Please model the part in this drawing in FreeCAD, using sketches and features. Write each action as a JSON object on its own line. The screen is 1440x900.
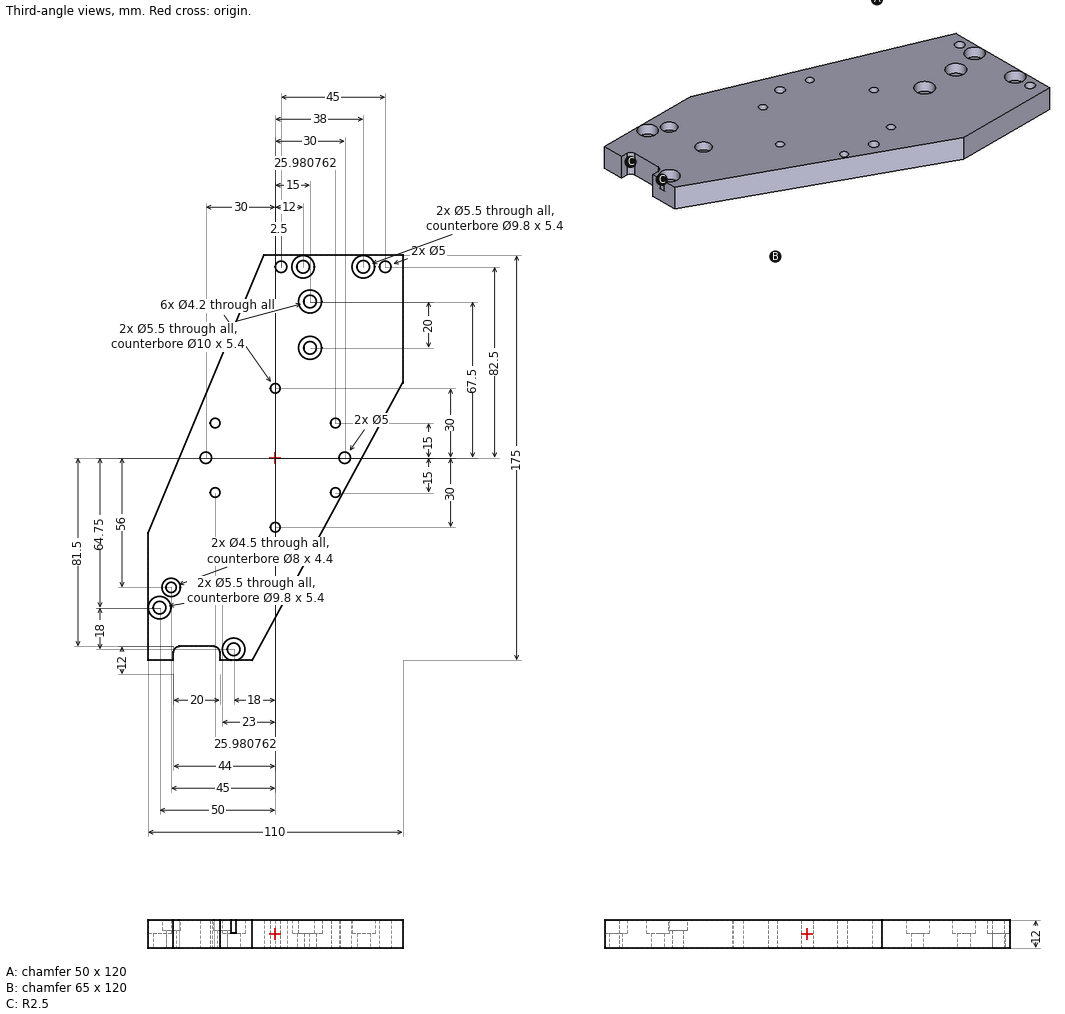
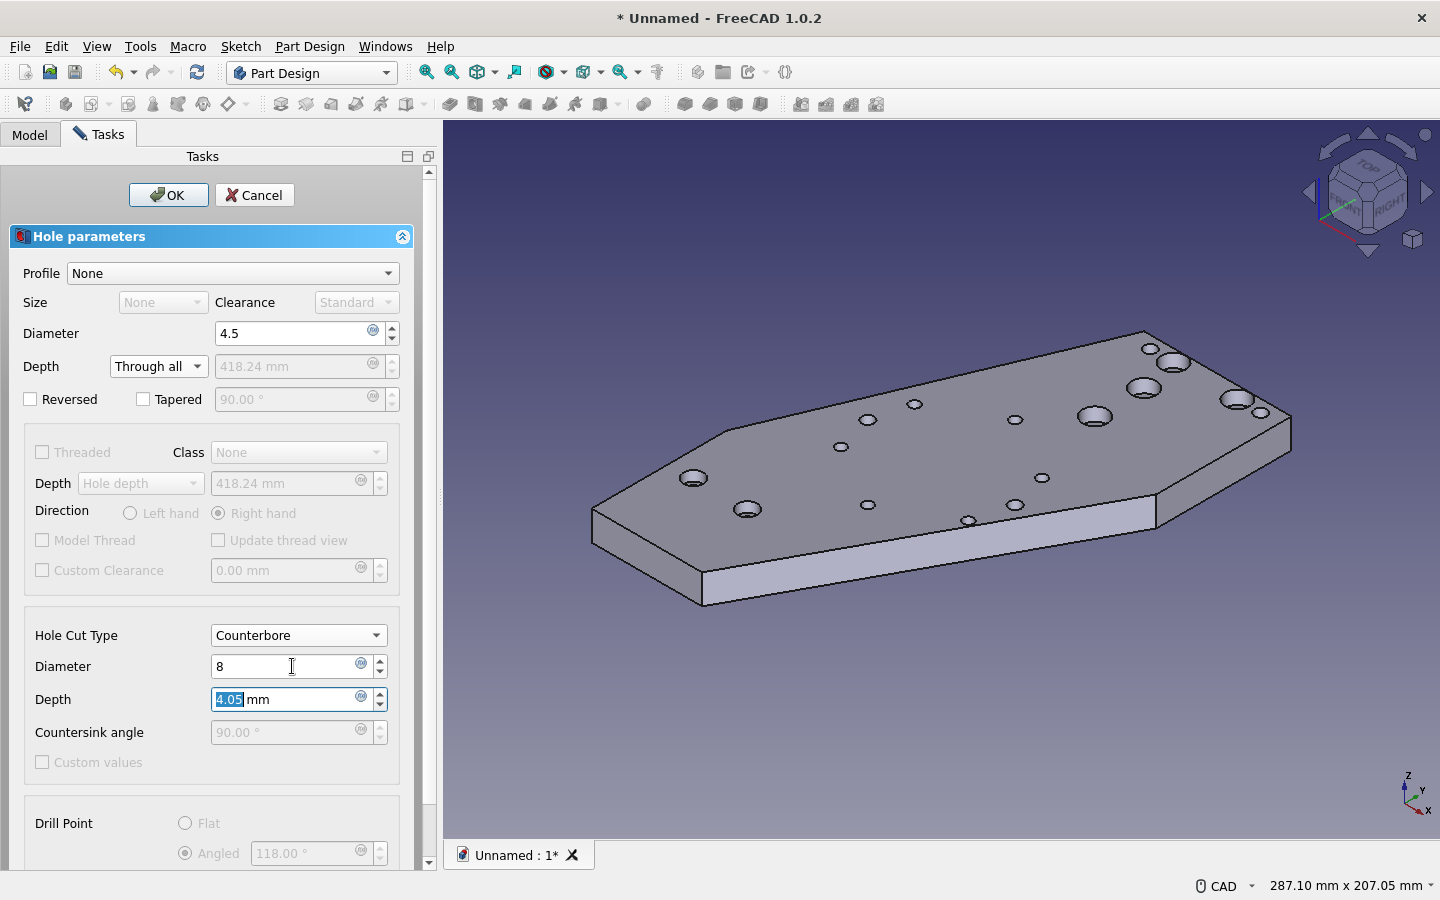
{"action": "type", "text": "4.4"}
{"action": "key", "text": "Tab"}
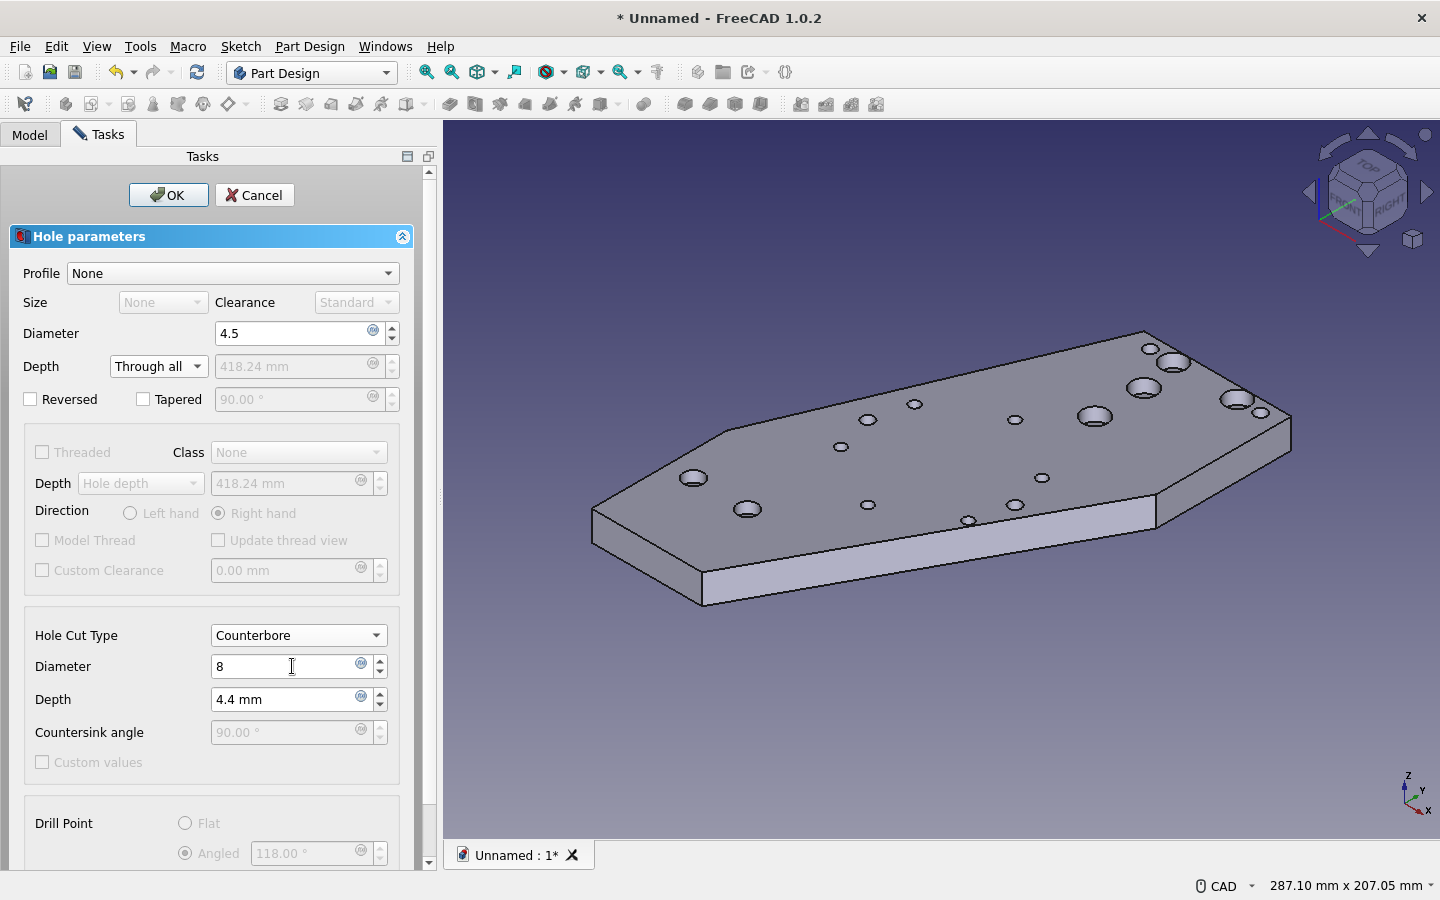
{"action": "left_click", "coordinate": [169, 195]}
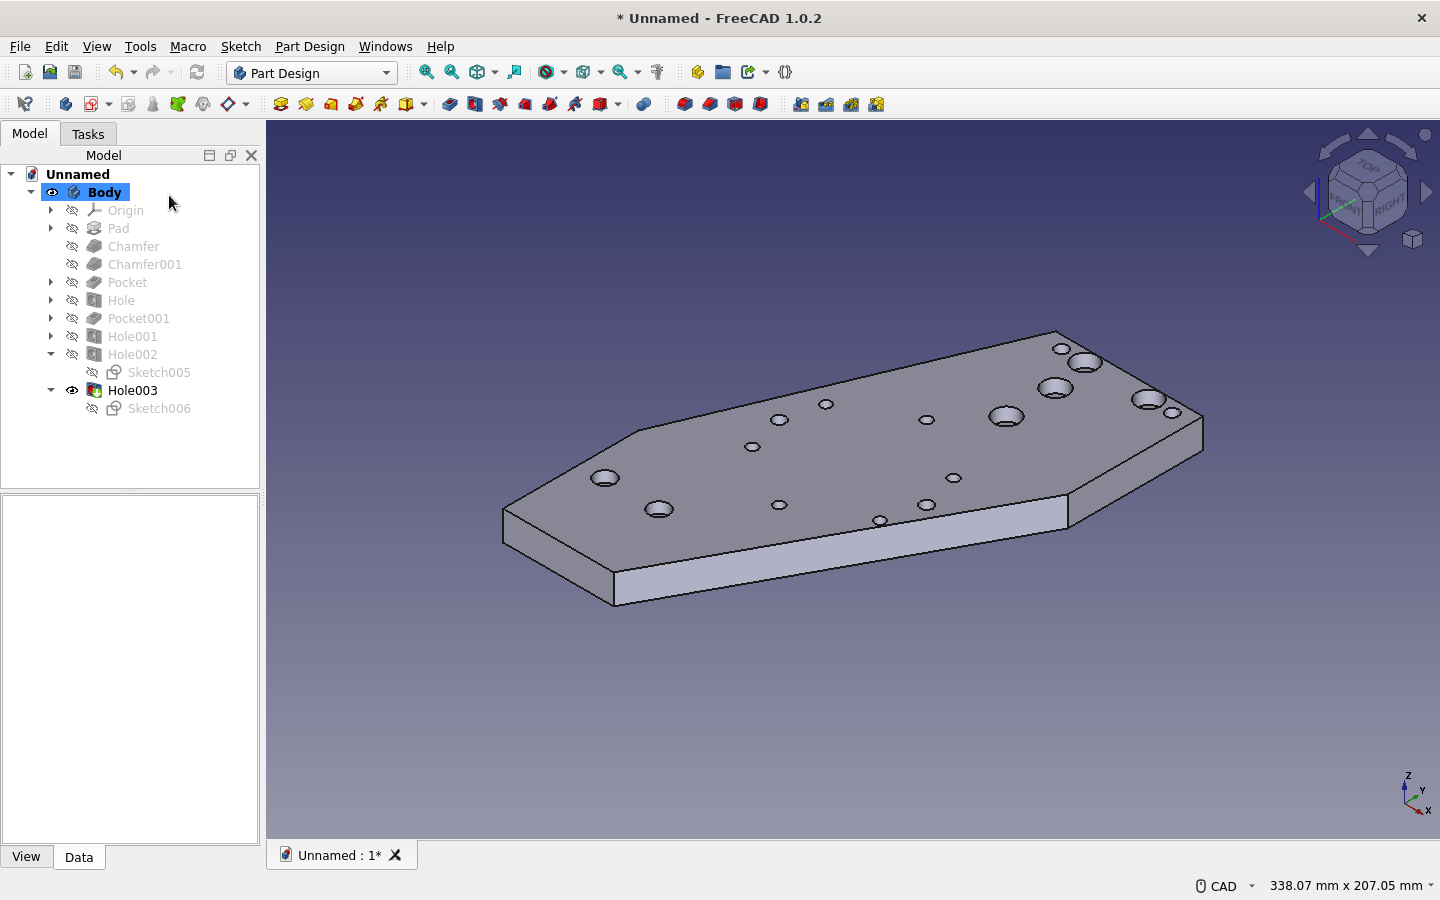
{"action": "left_click", "coordinate": [853, 461]}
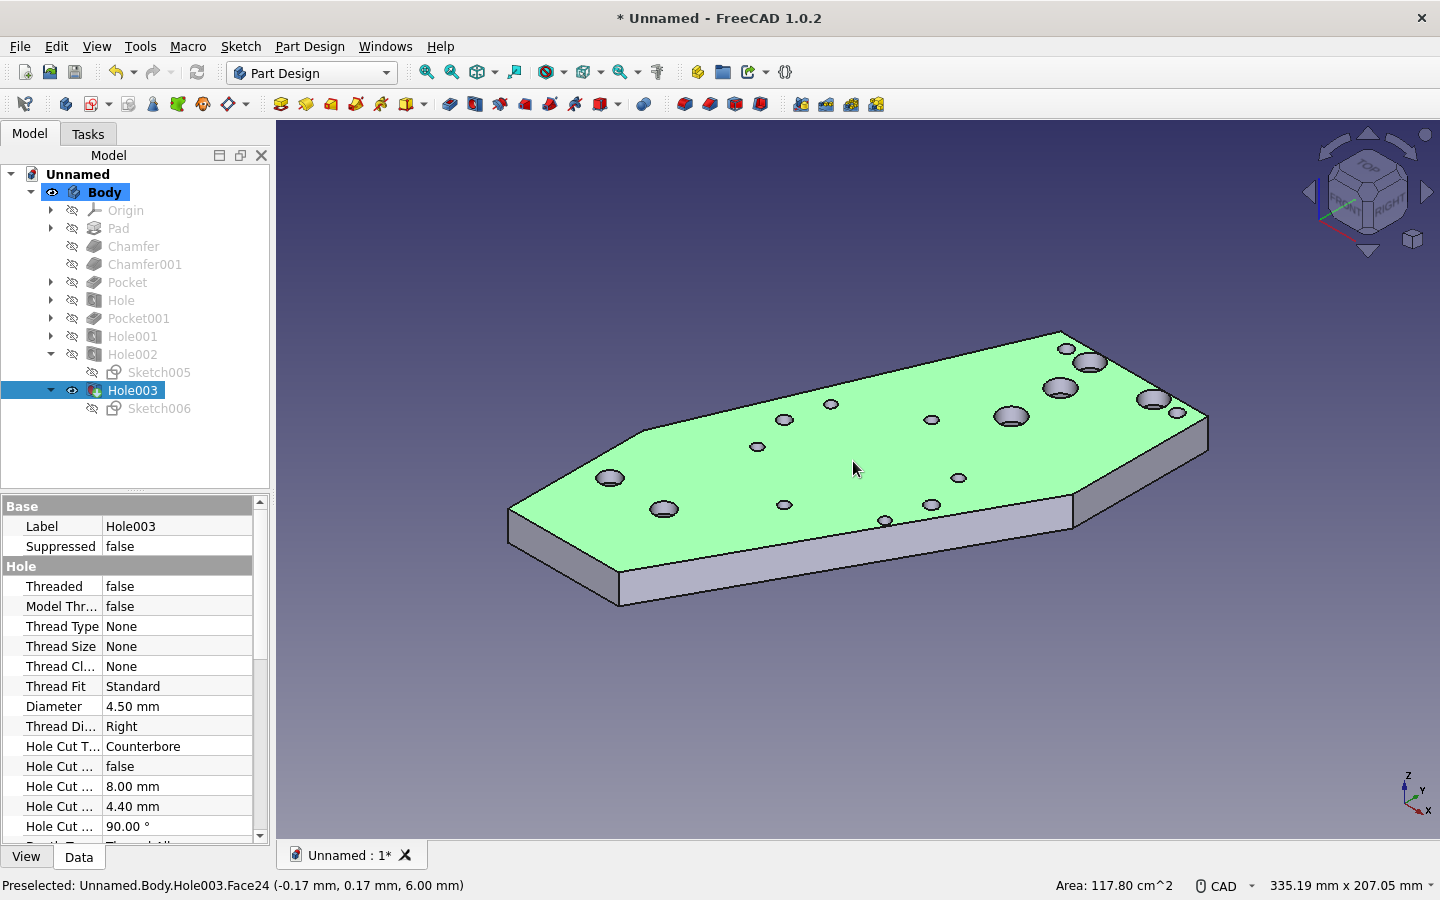
{"action": "left_click", "coordinate": [90, 104]}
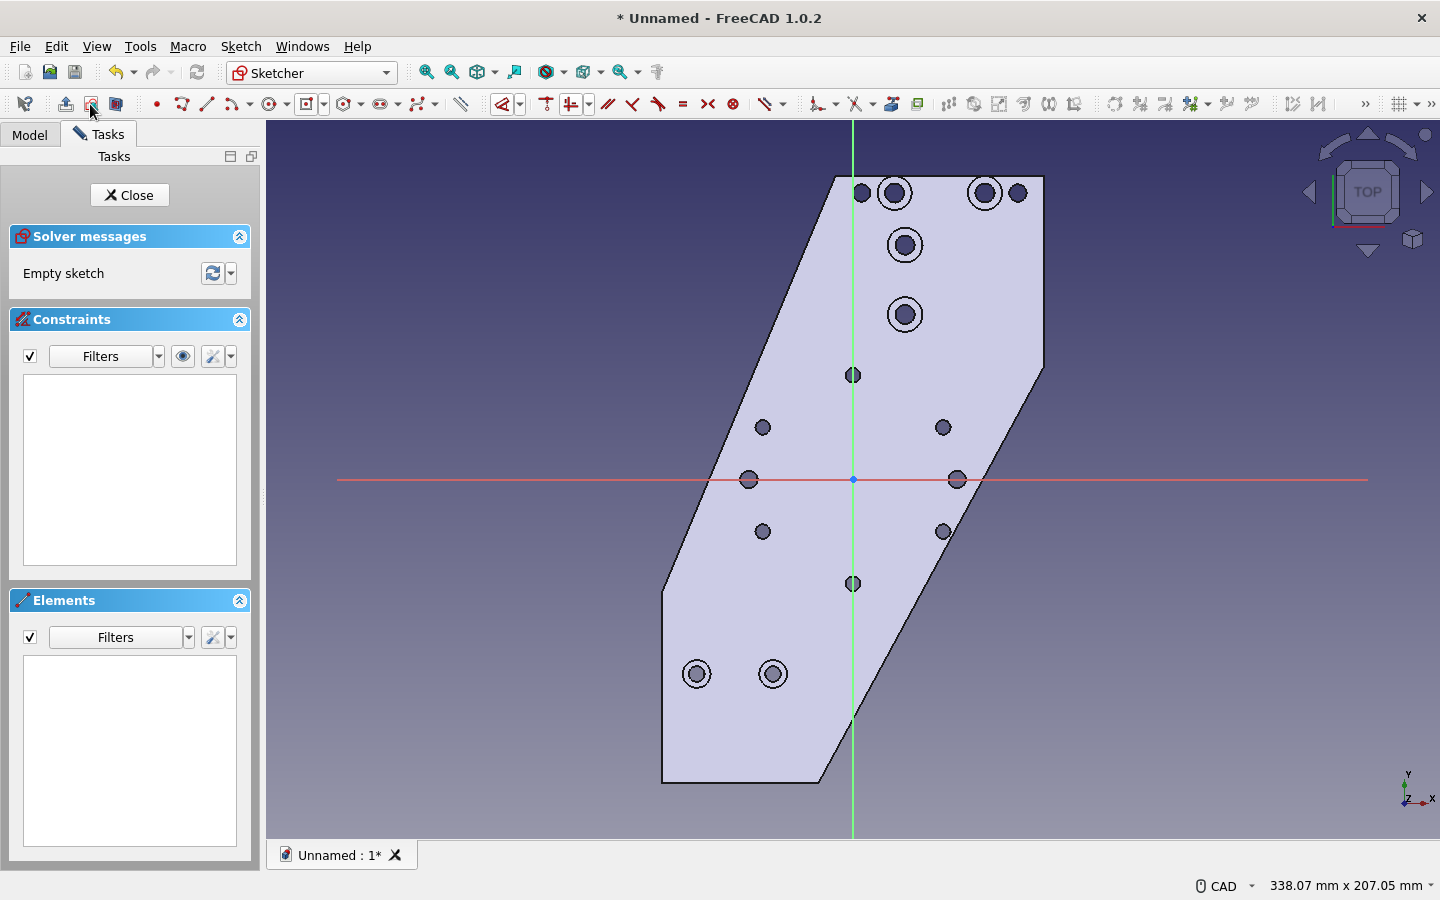
{"action": "scroll", "coordinate": [714, 811], "scroll_direction": "up", "scroll_amount": 2}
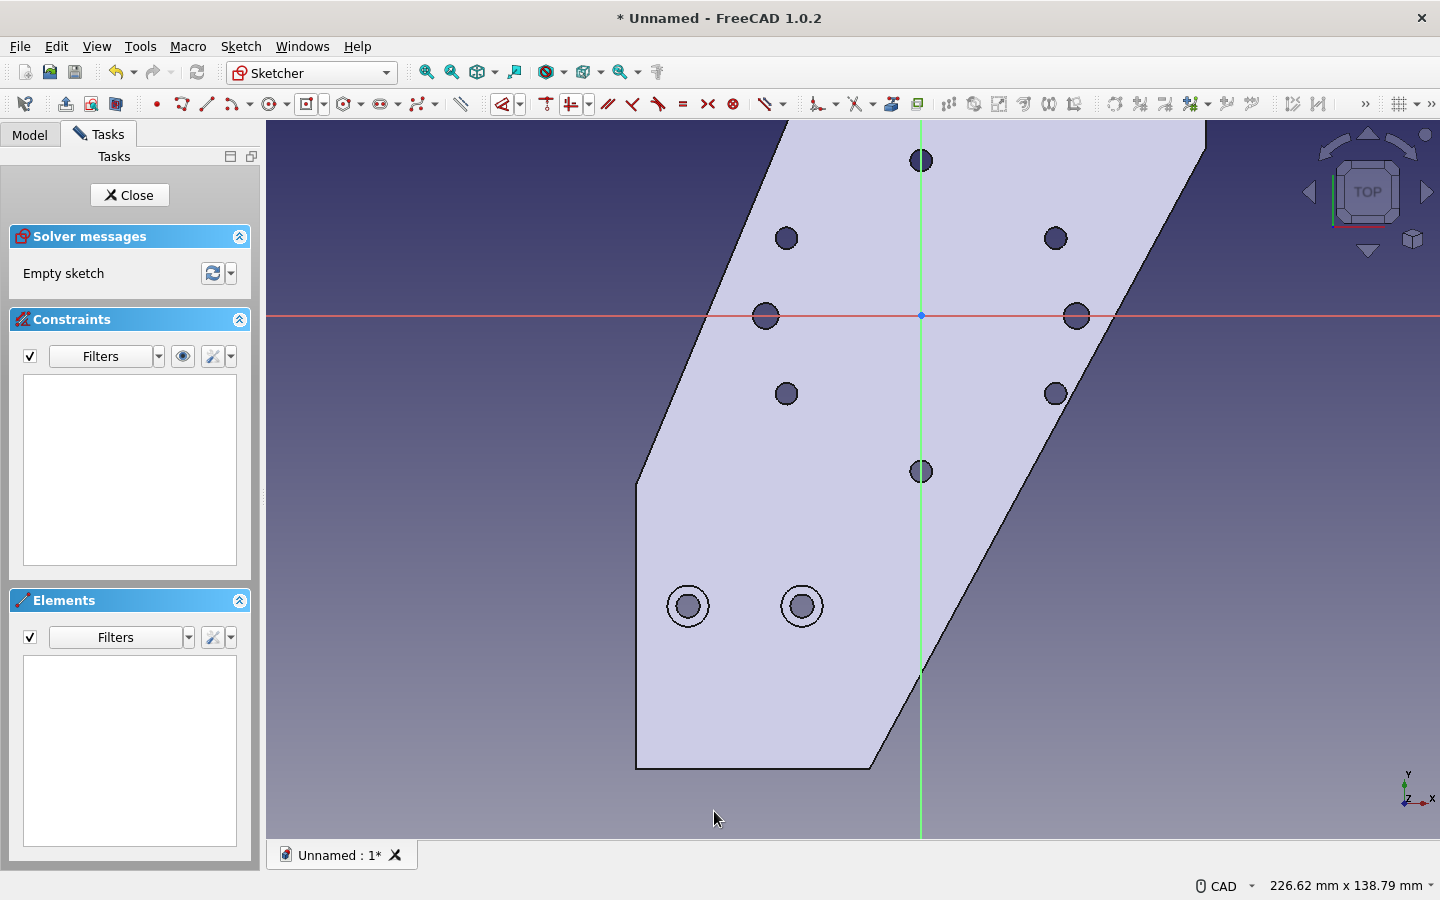
{"action": "key", "text": "g c"}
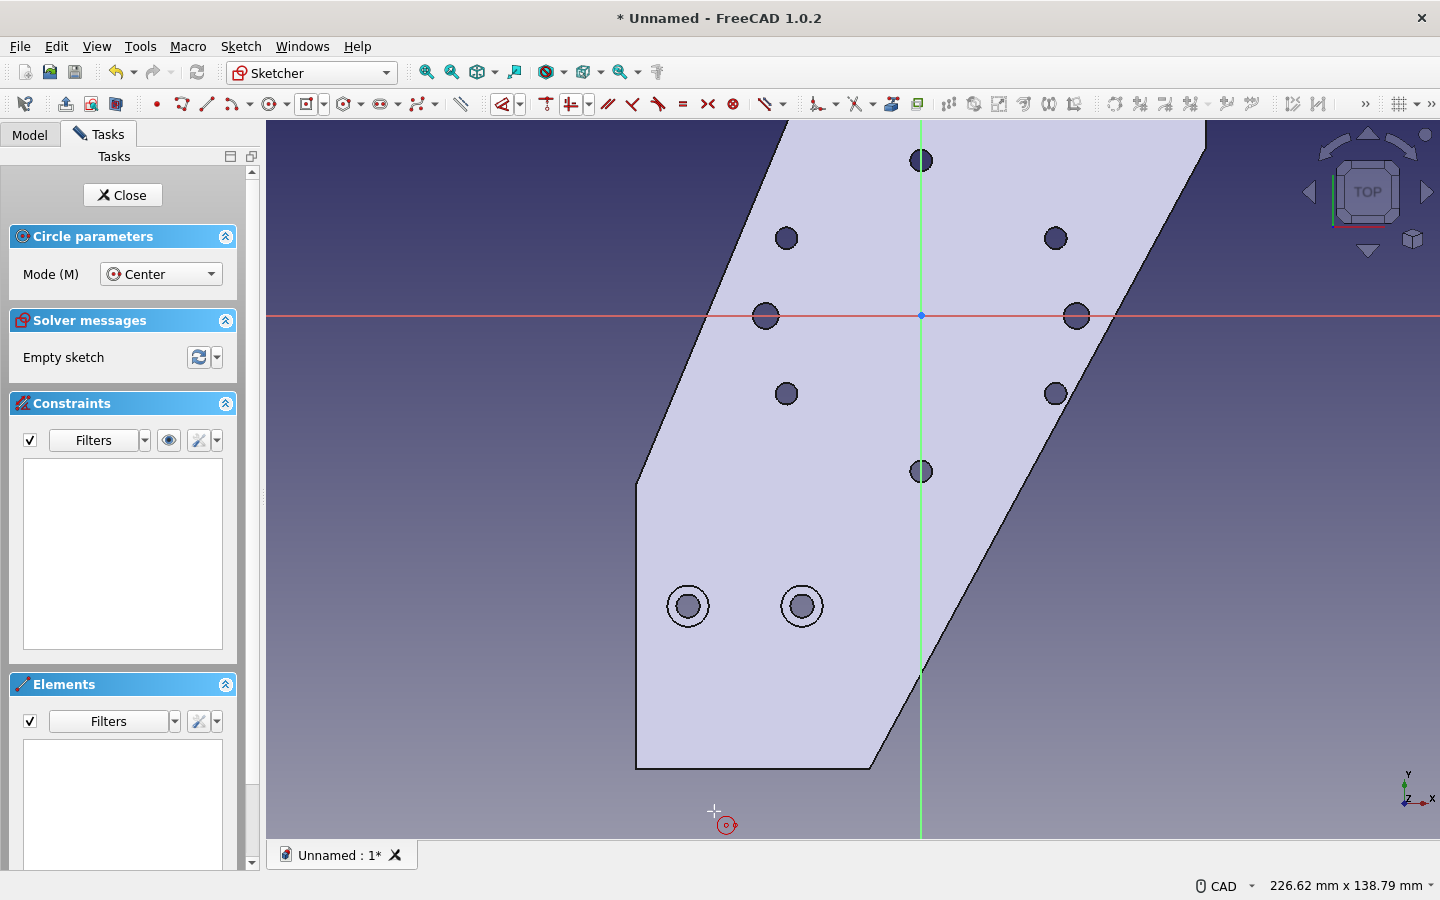
{"action": "scroll", "coordinate": [662, 651], "scroll_direction": "up", "scroll_amount": 3}